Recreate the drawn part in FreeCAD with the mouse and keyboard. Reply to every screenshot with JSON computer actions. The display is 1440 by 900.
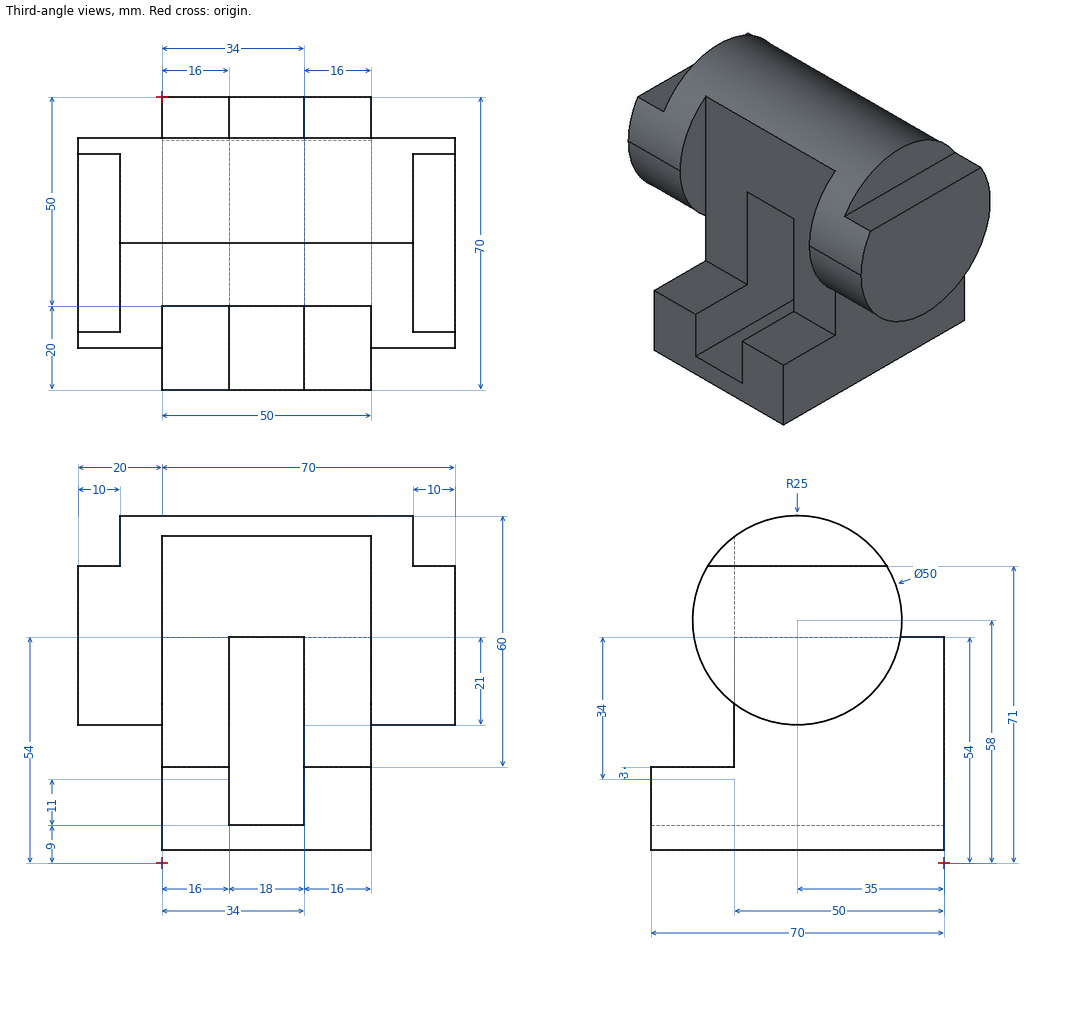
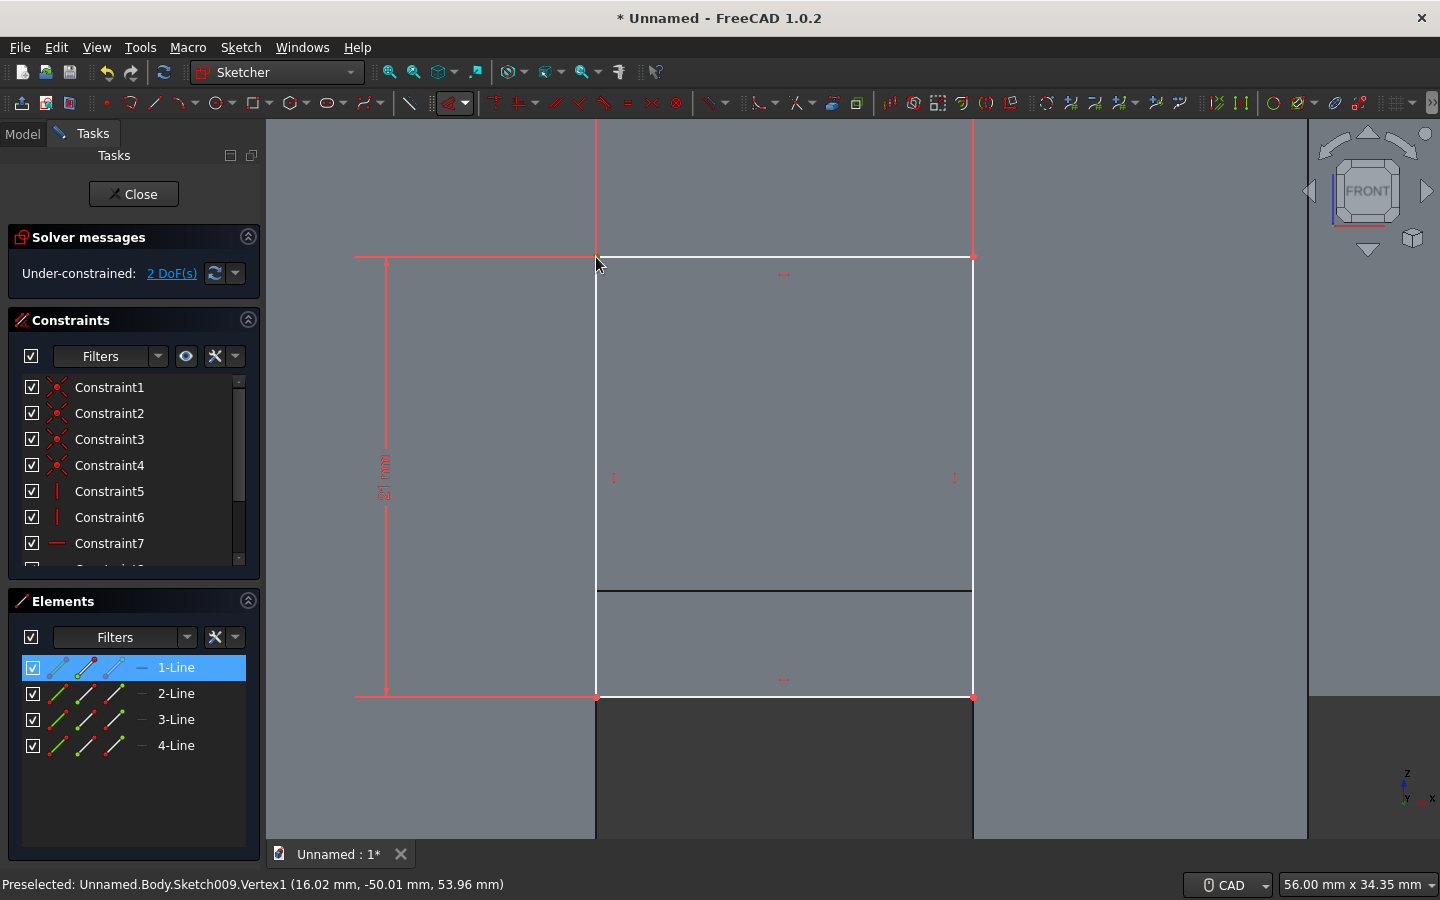
{"action": "key", "text": "l"}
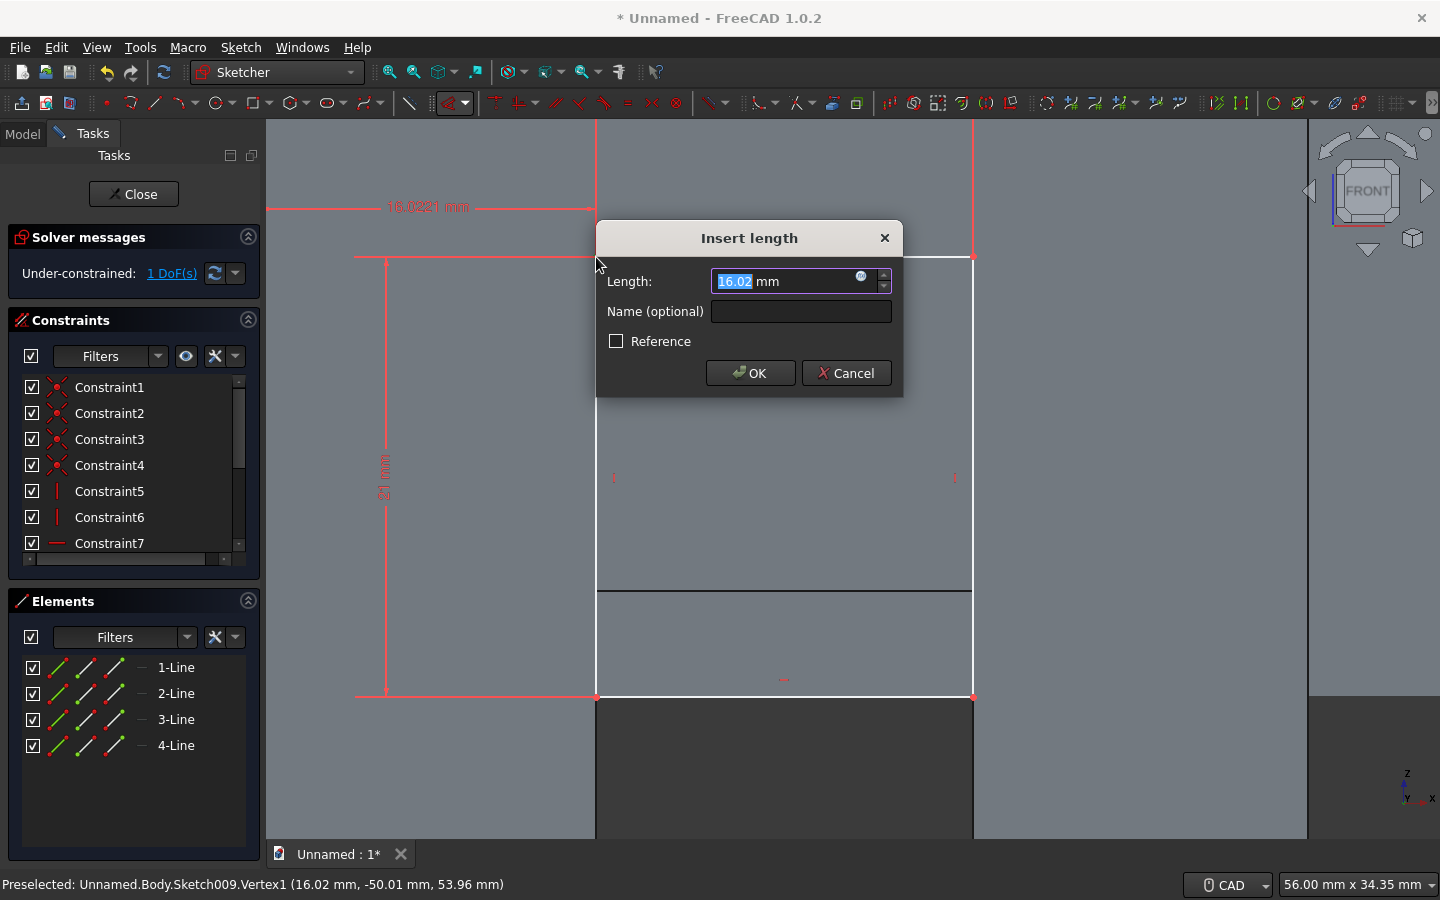
{"action": "type", "text": "16"}
{"action": "key", "text": "Return"}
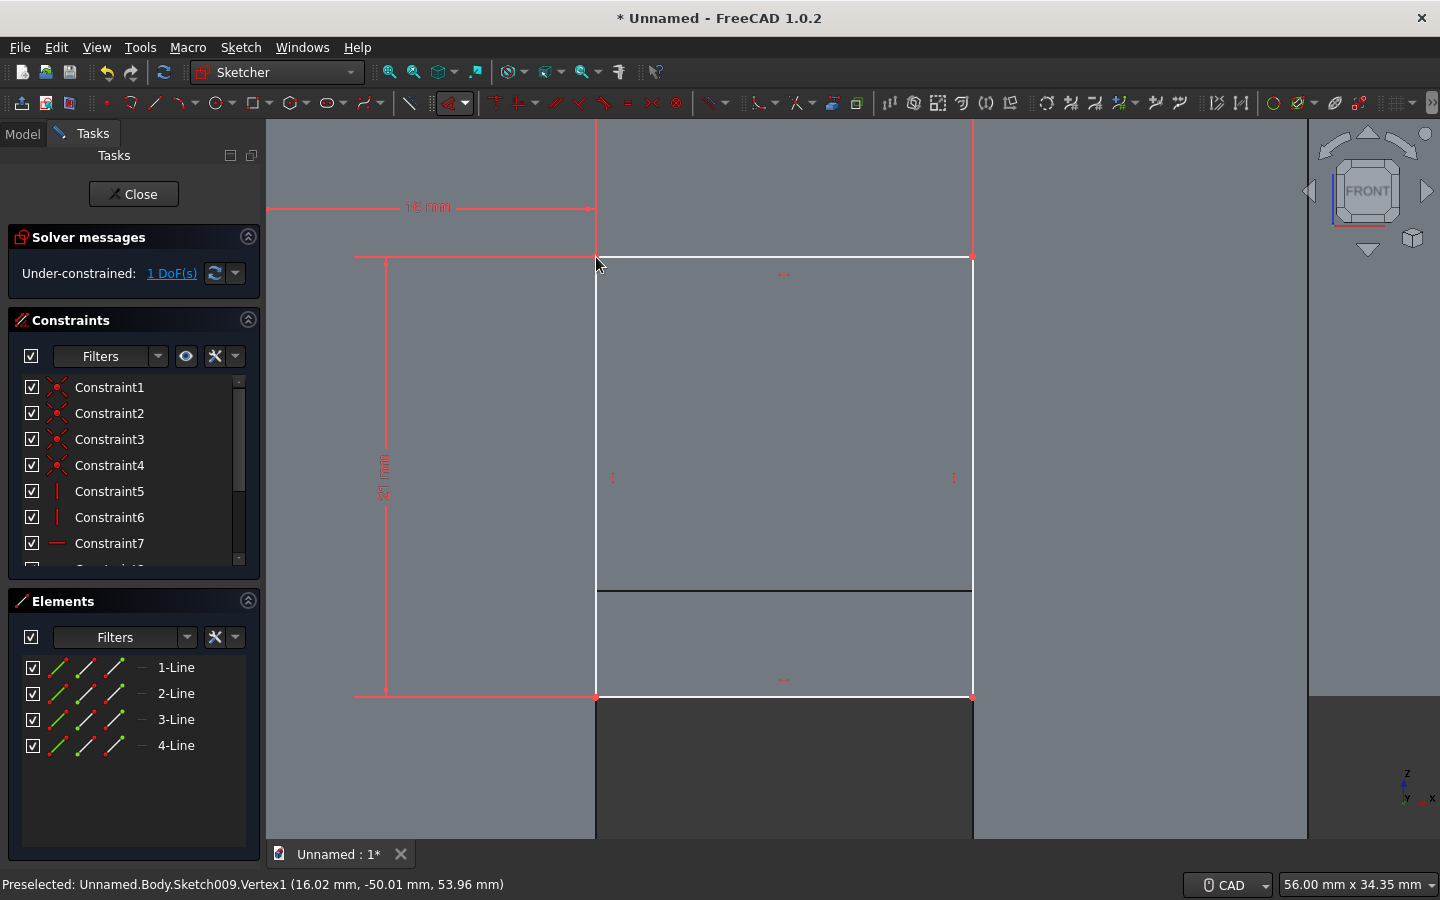
{"action": "left_click", "coordinate": [596, 257]}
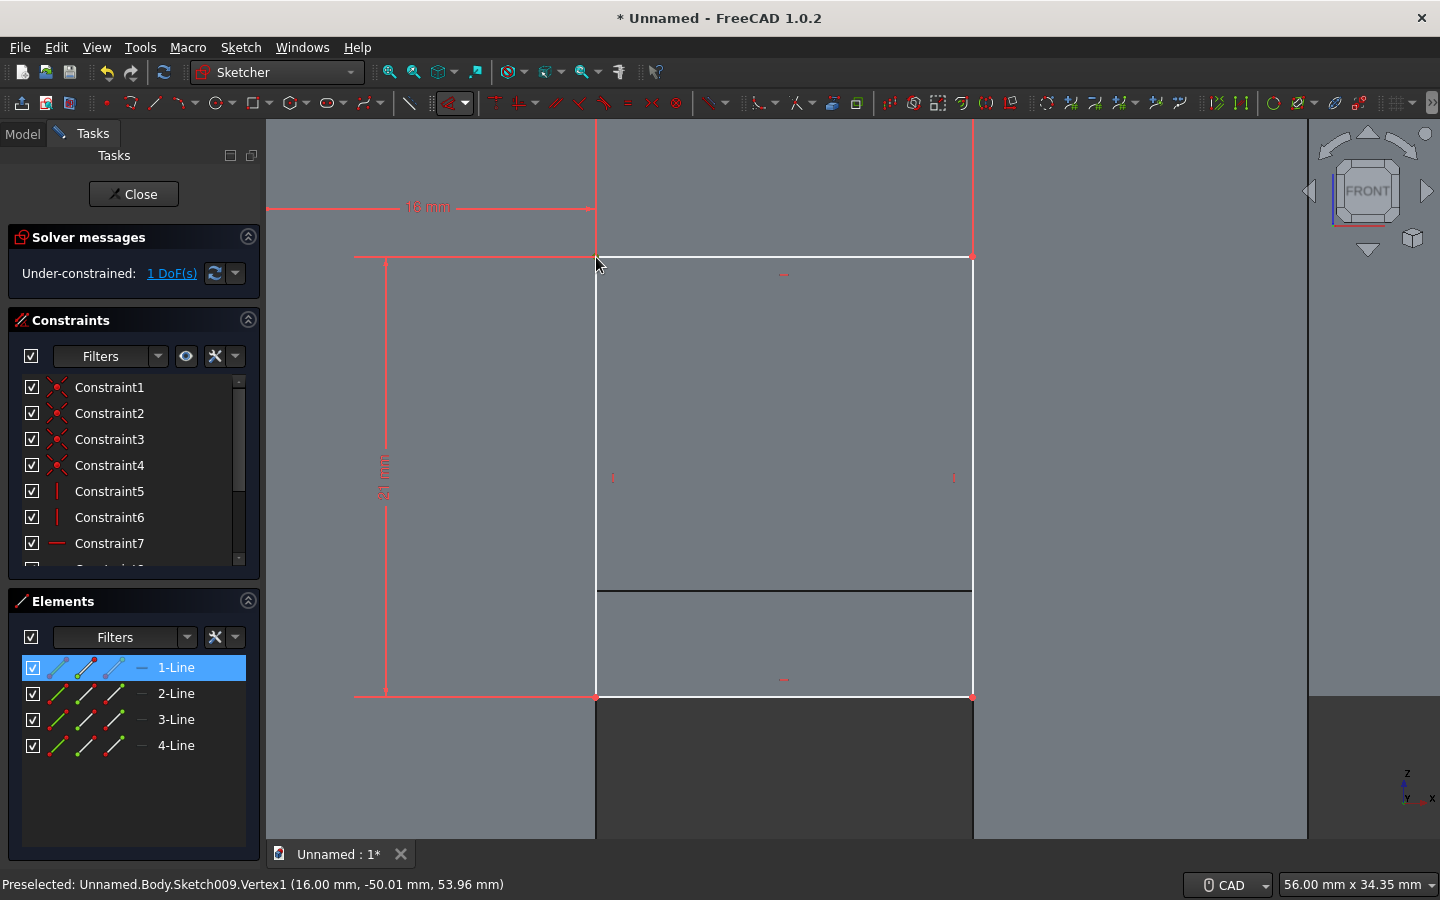
{"action": "left_click", "coordinate": [468, 104]}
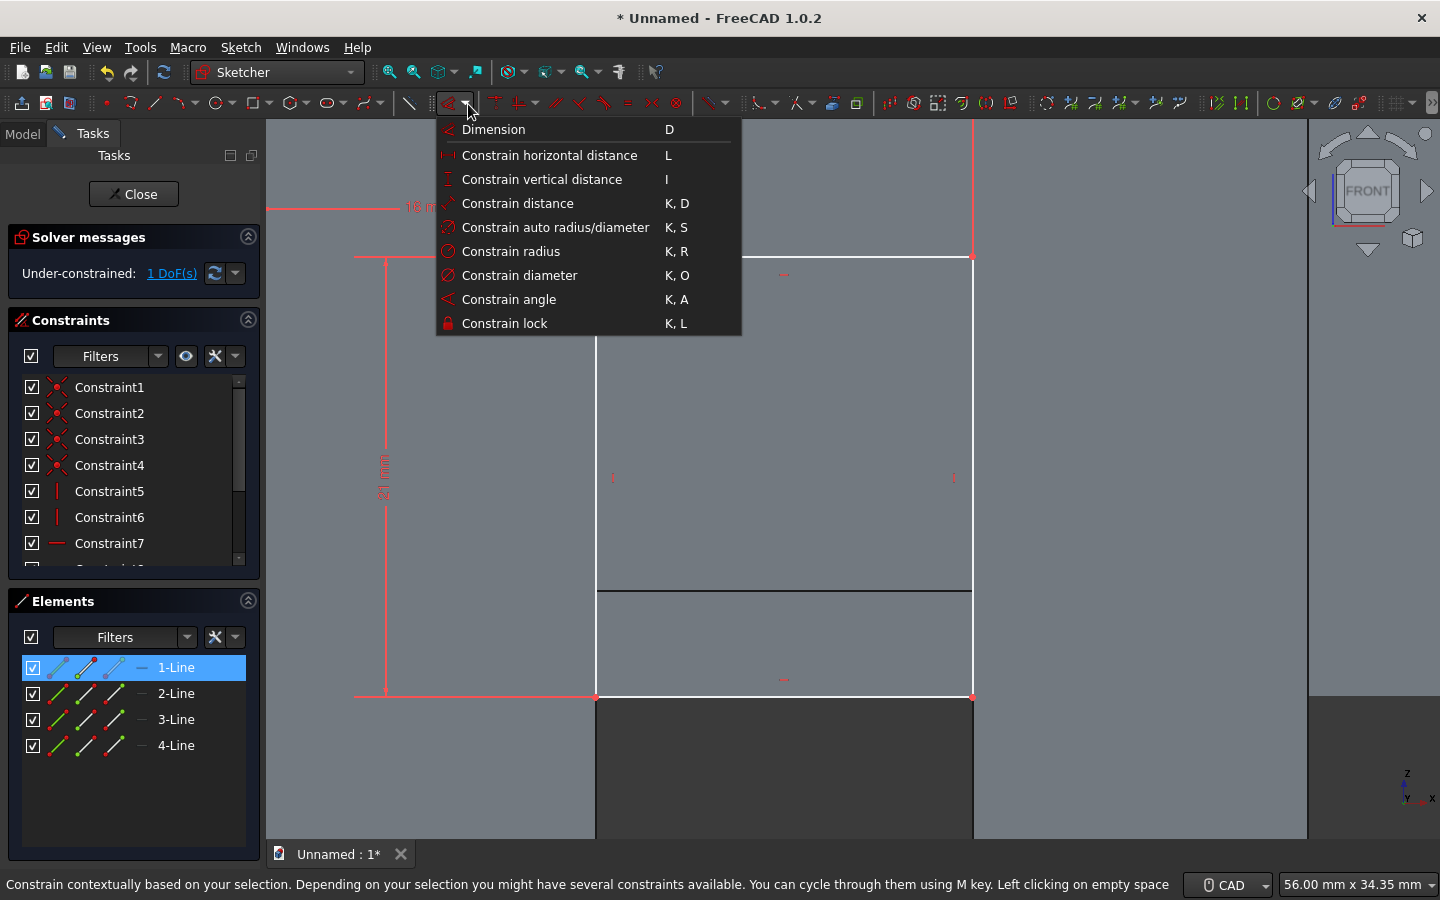
{"action": "left_click", "coordinate": [589, 179]}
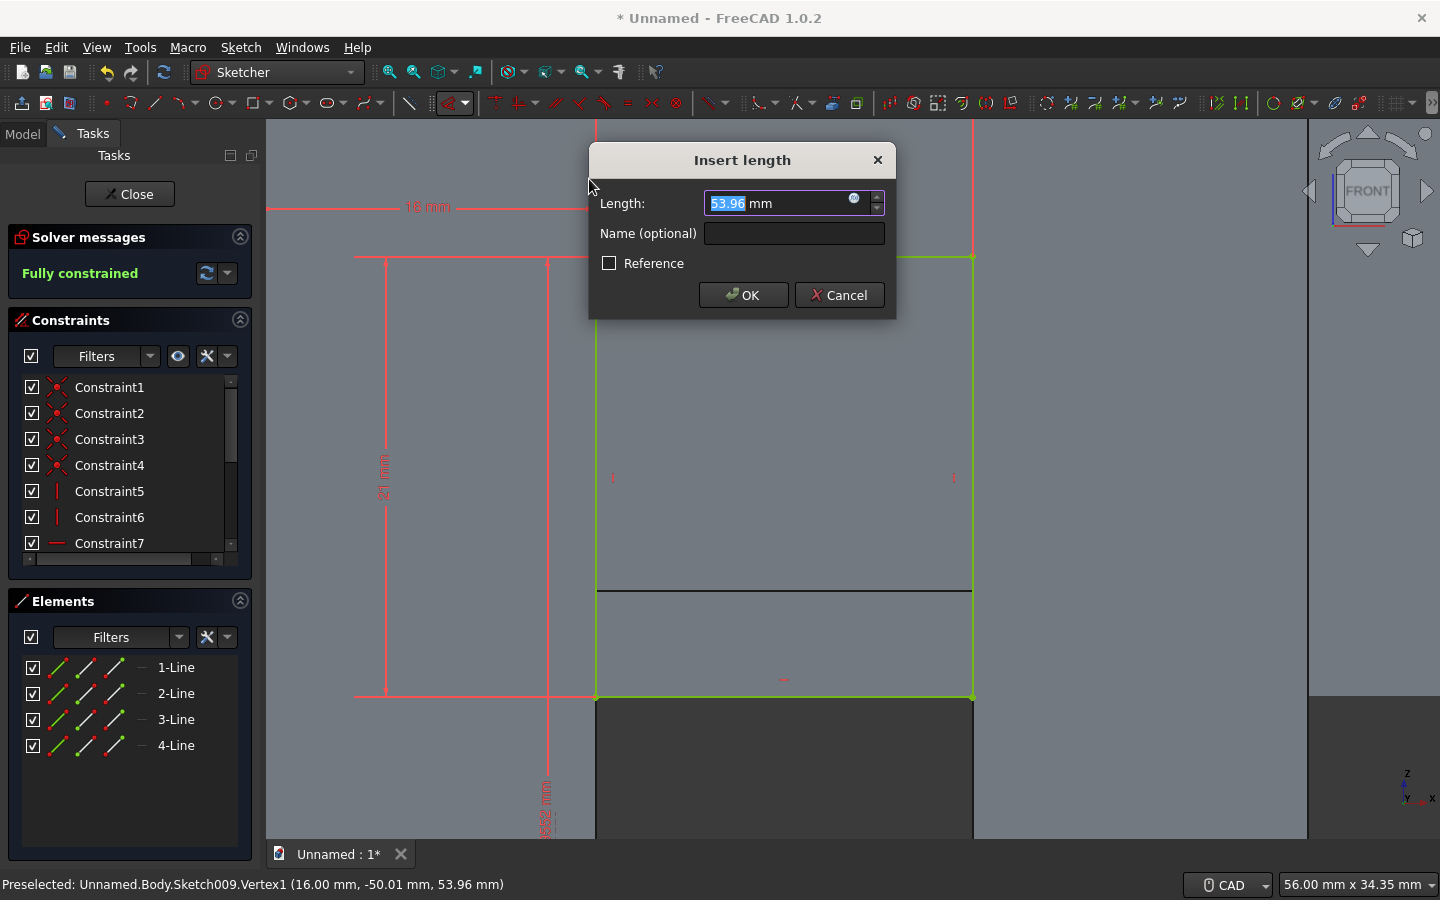
{"action": "type", "text": "54"}
{"action": "key", "text": "Return"}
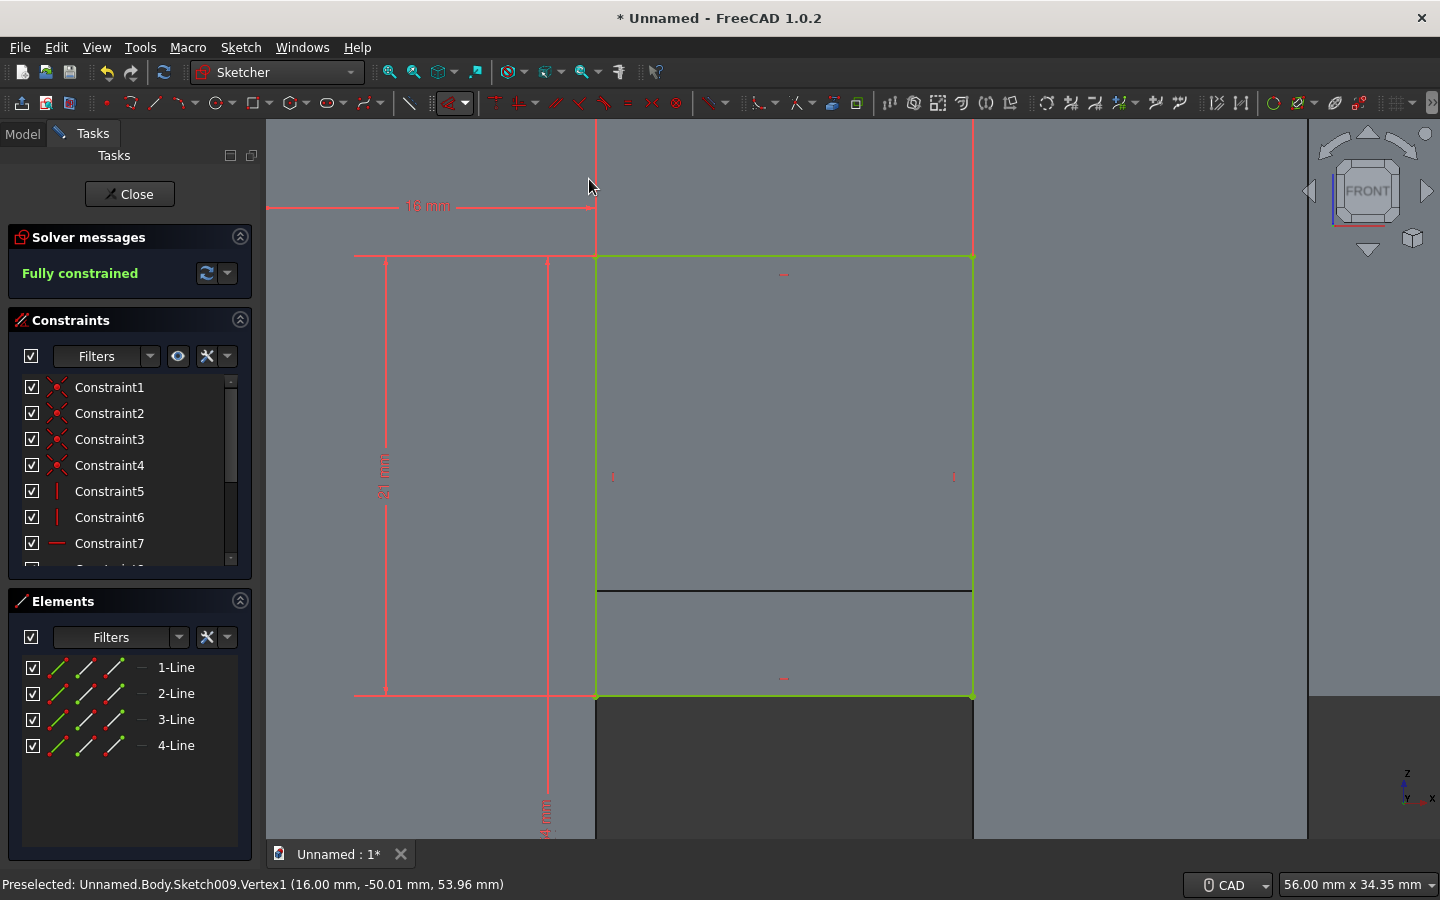
{"action": "left_click", "coordinate": [130, 194]}